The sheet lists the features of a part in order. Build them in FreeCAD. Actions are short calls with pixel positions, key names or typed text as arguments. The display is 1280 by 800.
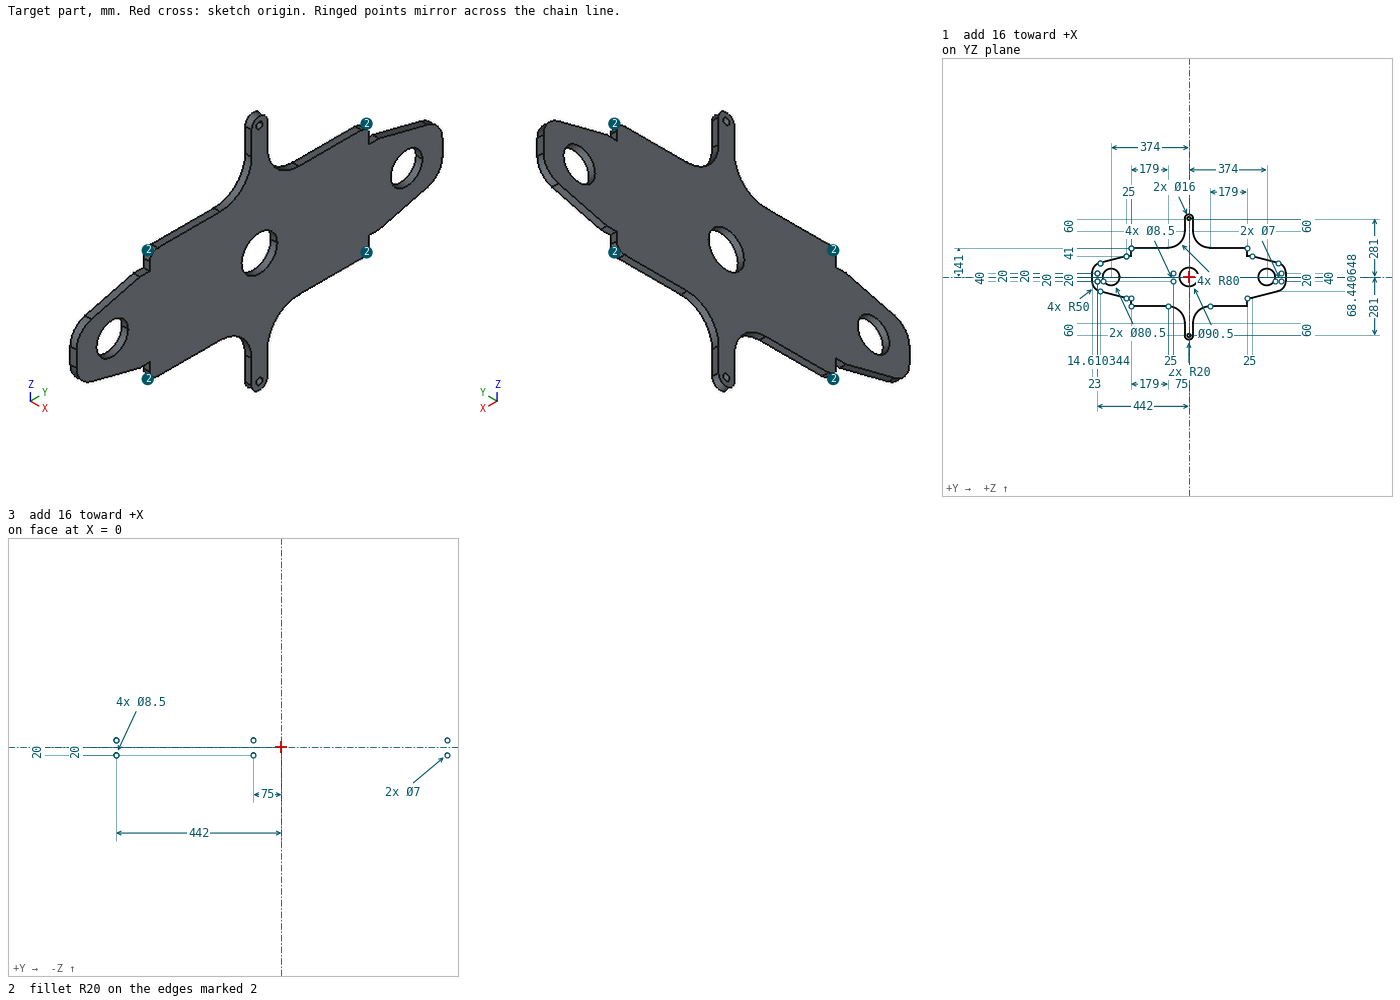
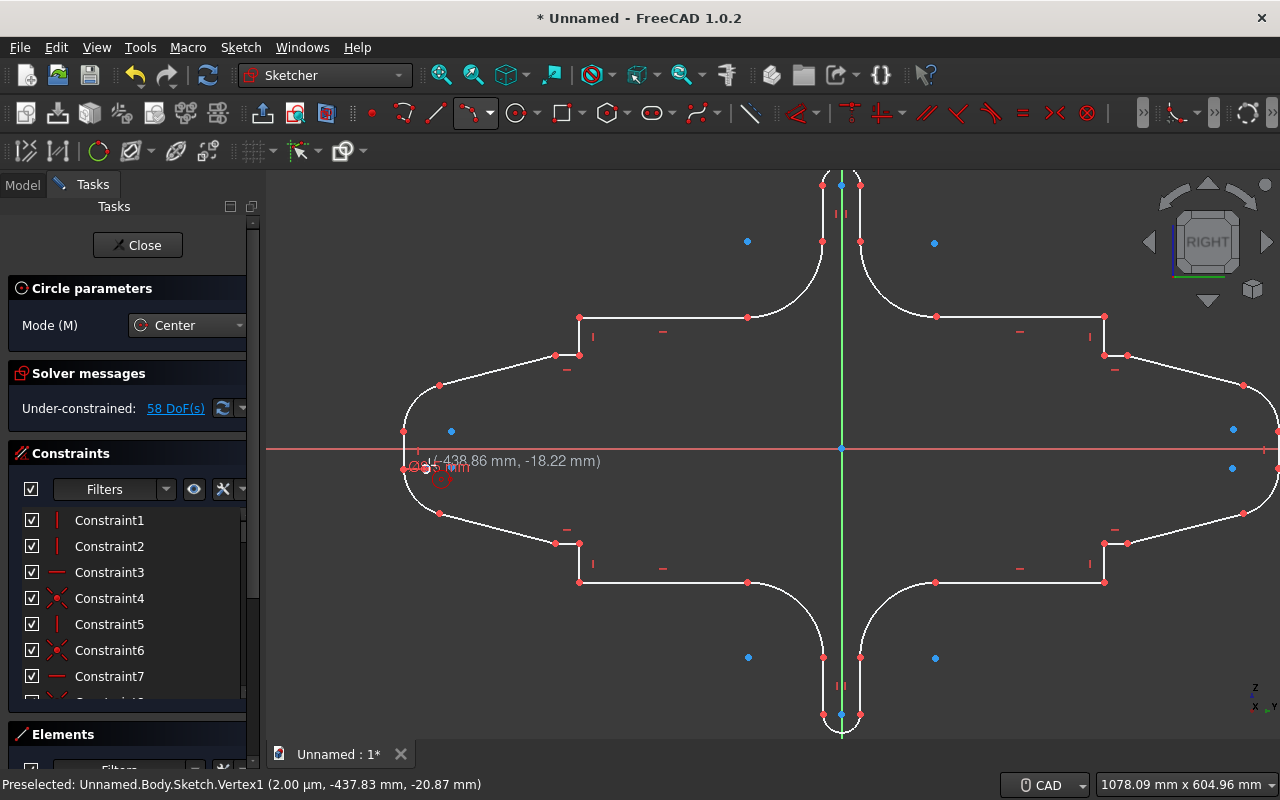
scroll(771, 468, up, 9)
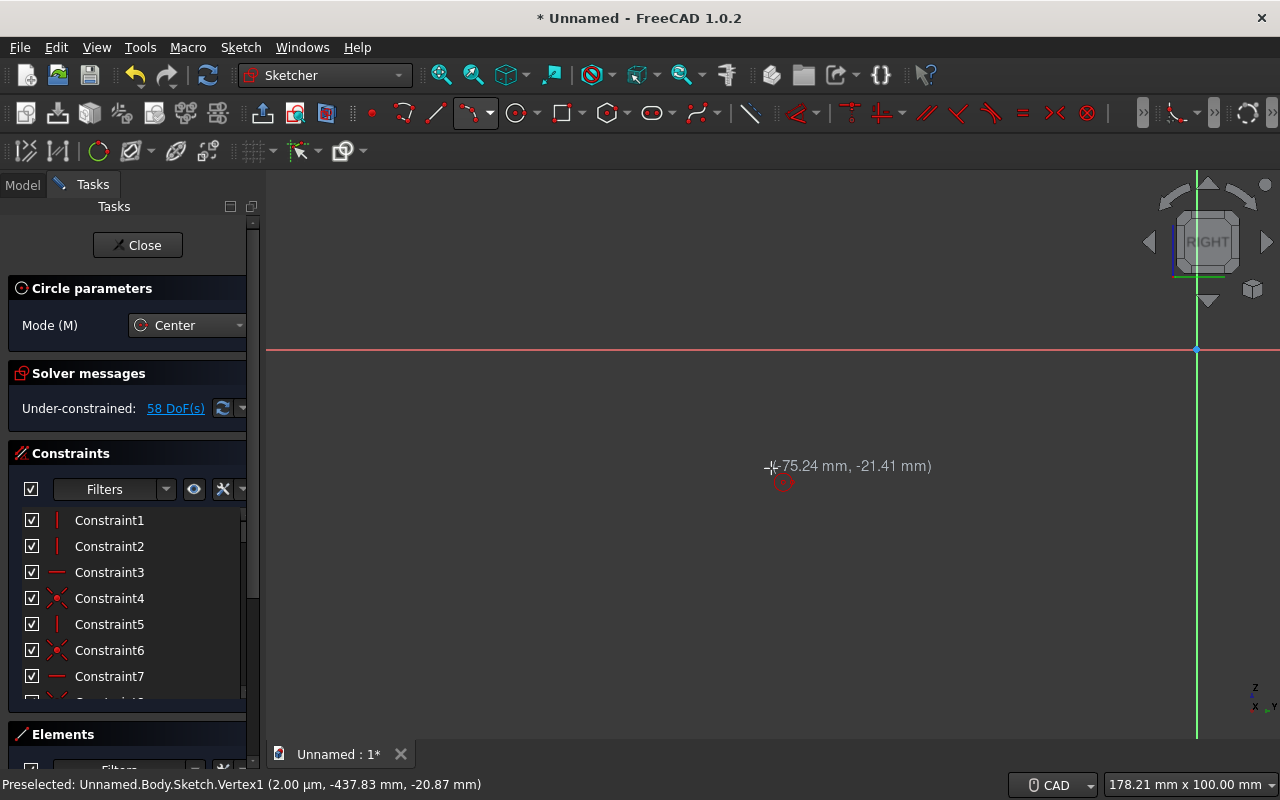
scroll(643, 468, down, 11)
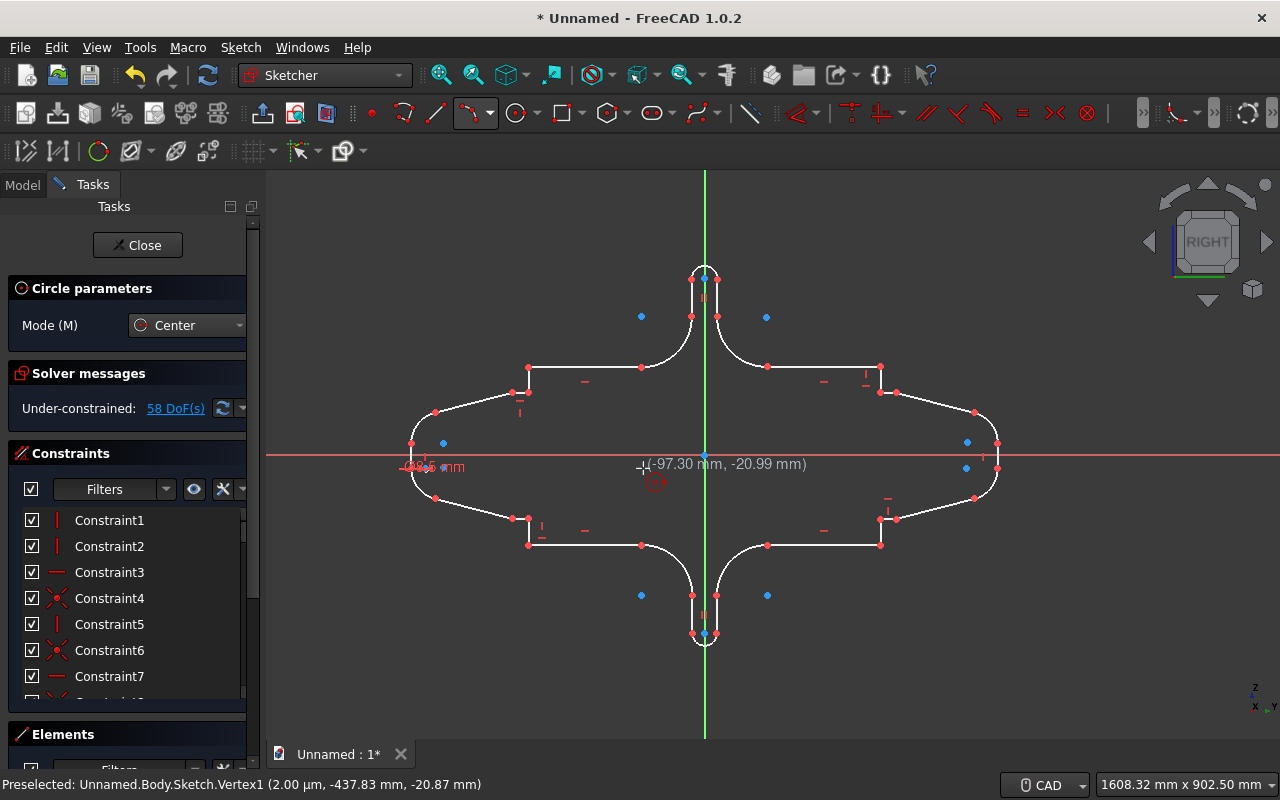
scroll(657, 468, up, 2)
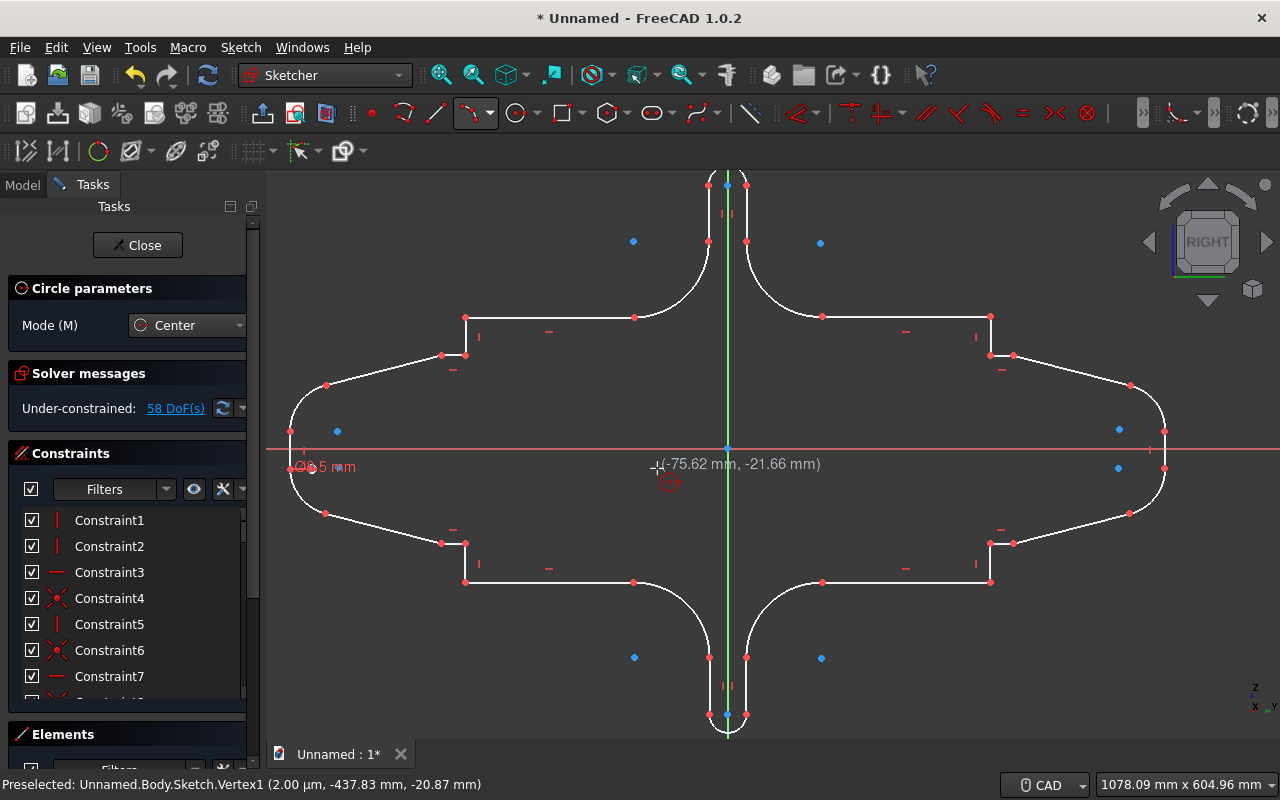
click(657, 468)
move(660, 465)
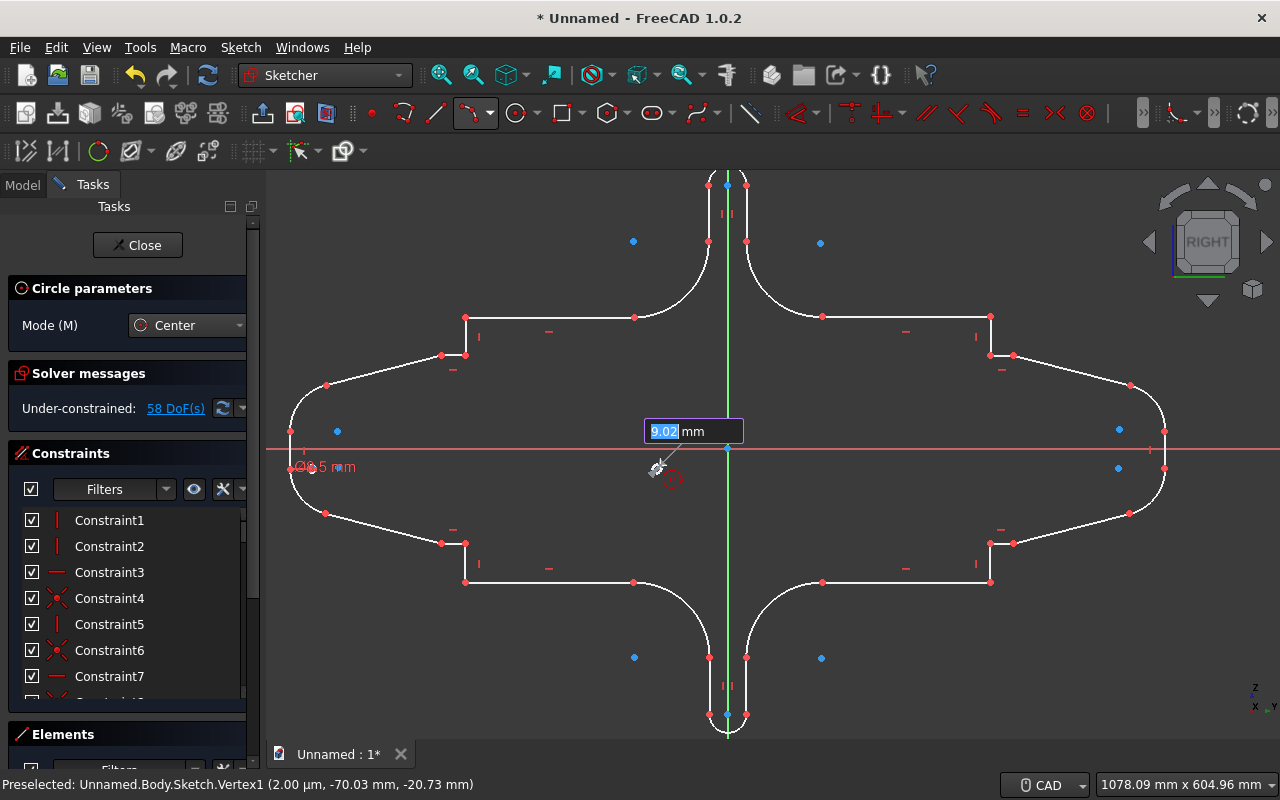
text(8.5)
key(Return)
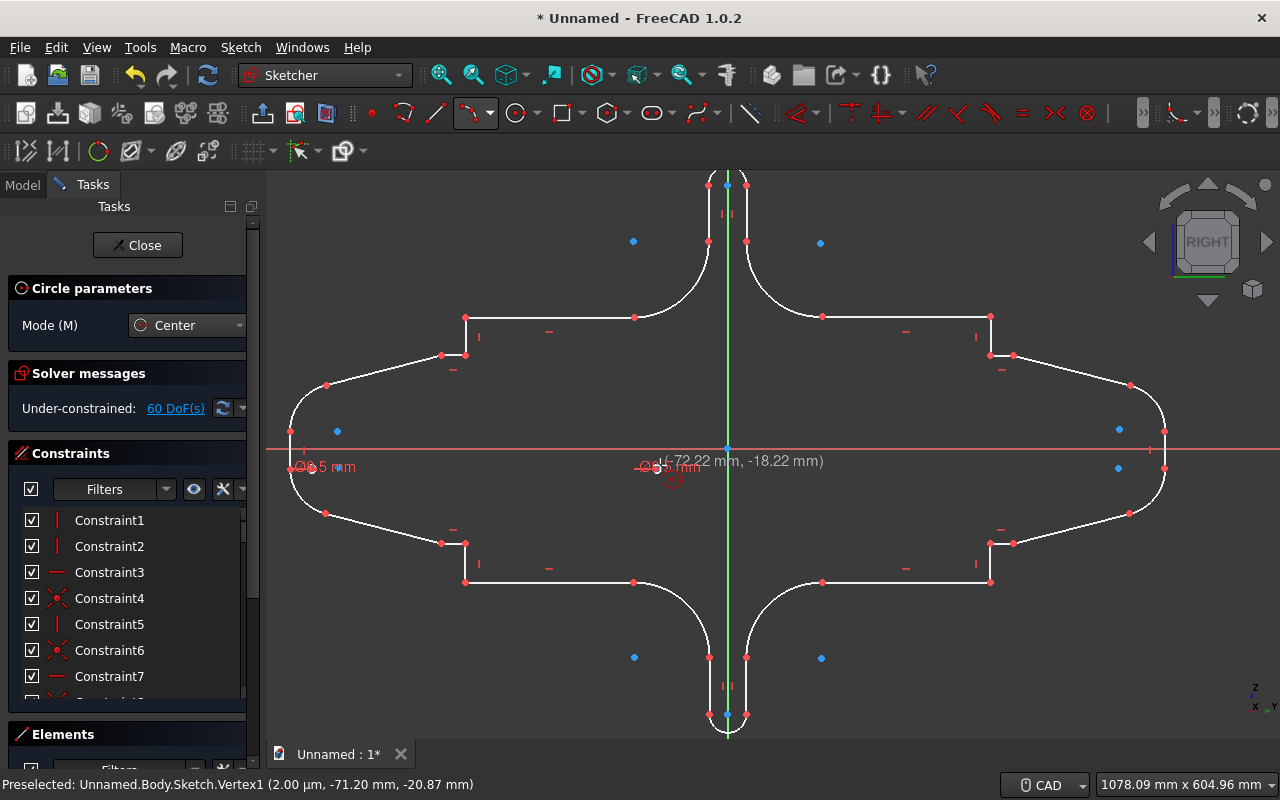
scroll(312, 430, up, 9)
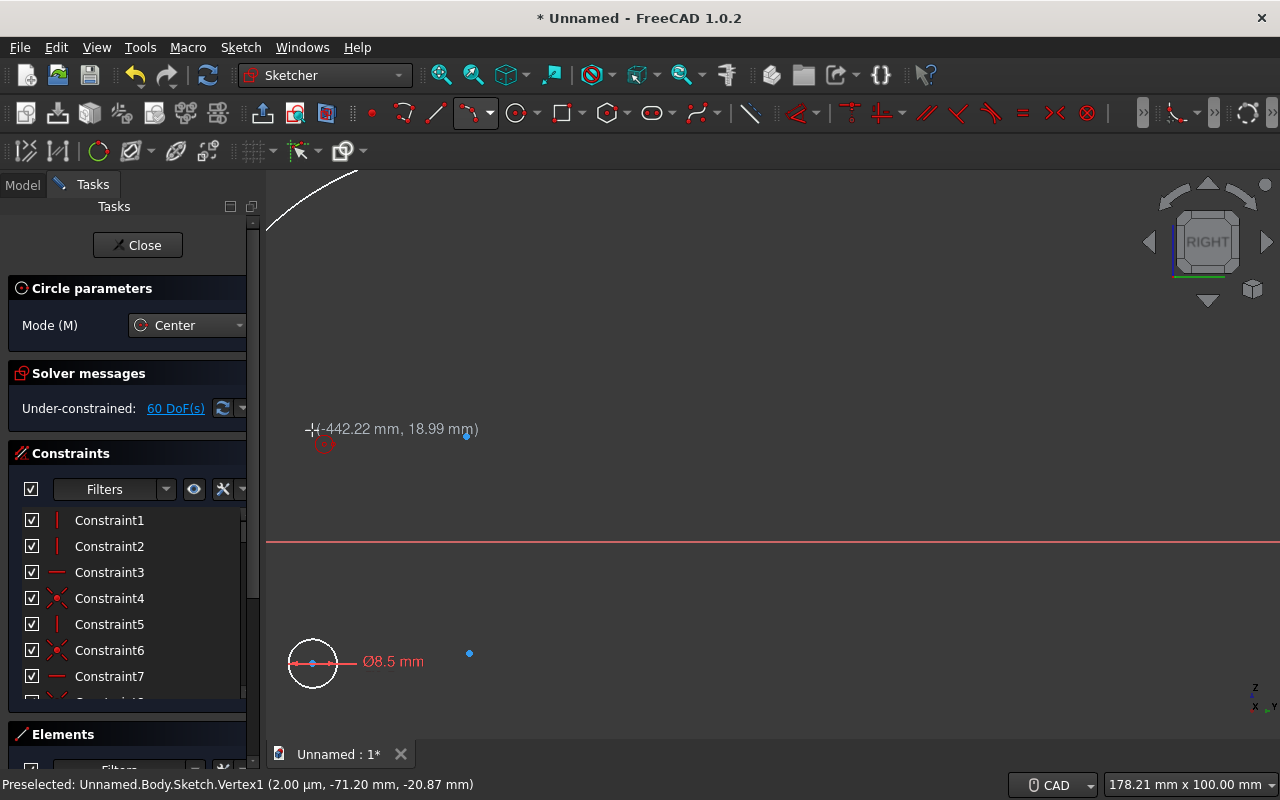
scroll(440, 444, down, 11)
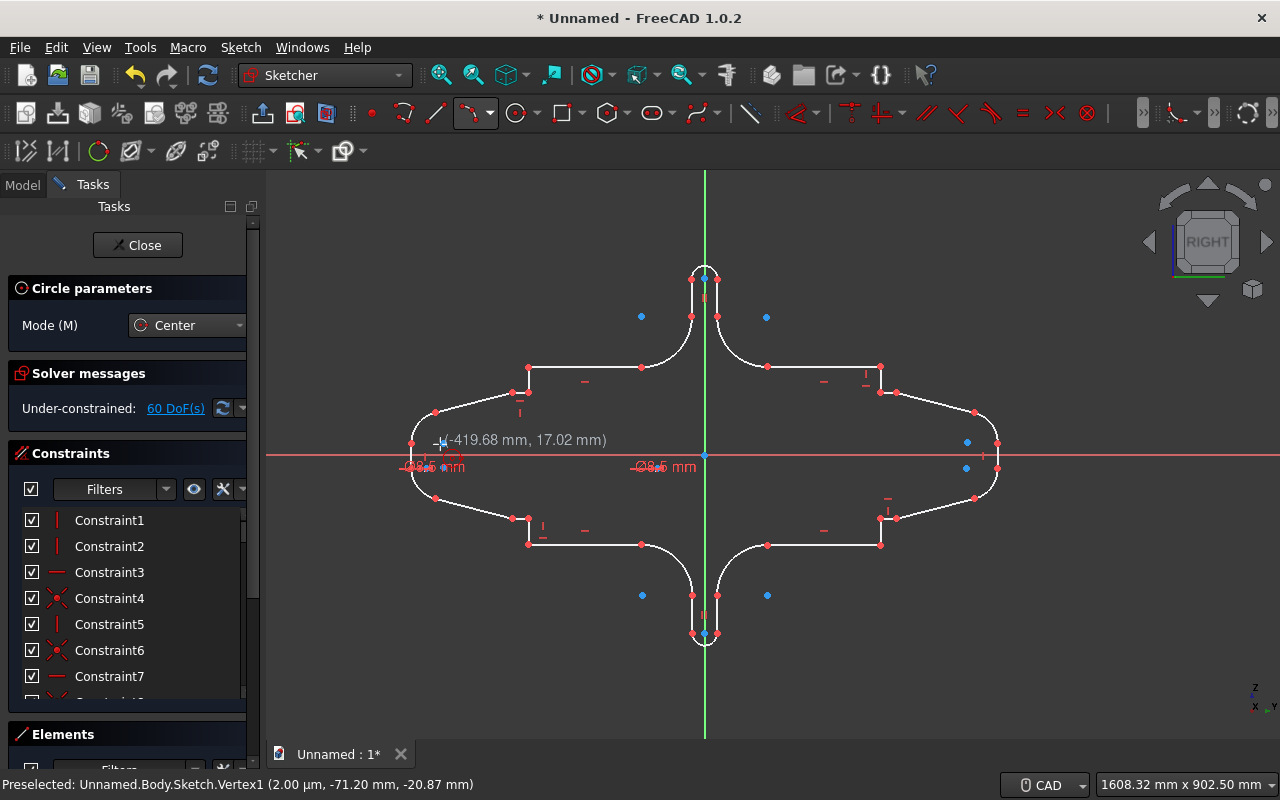
scroll(426, 443, up, 2)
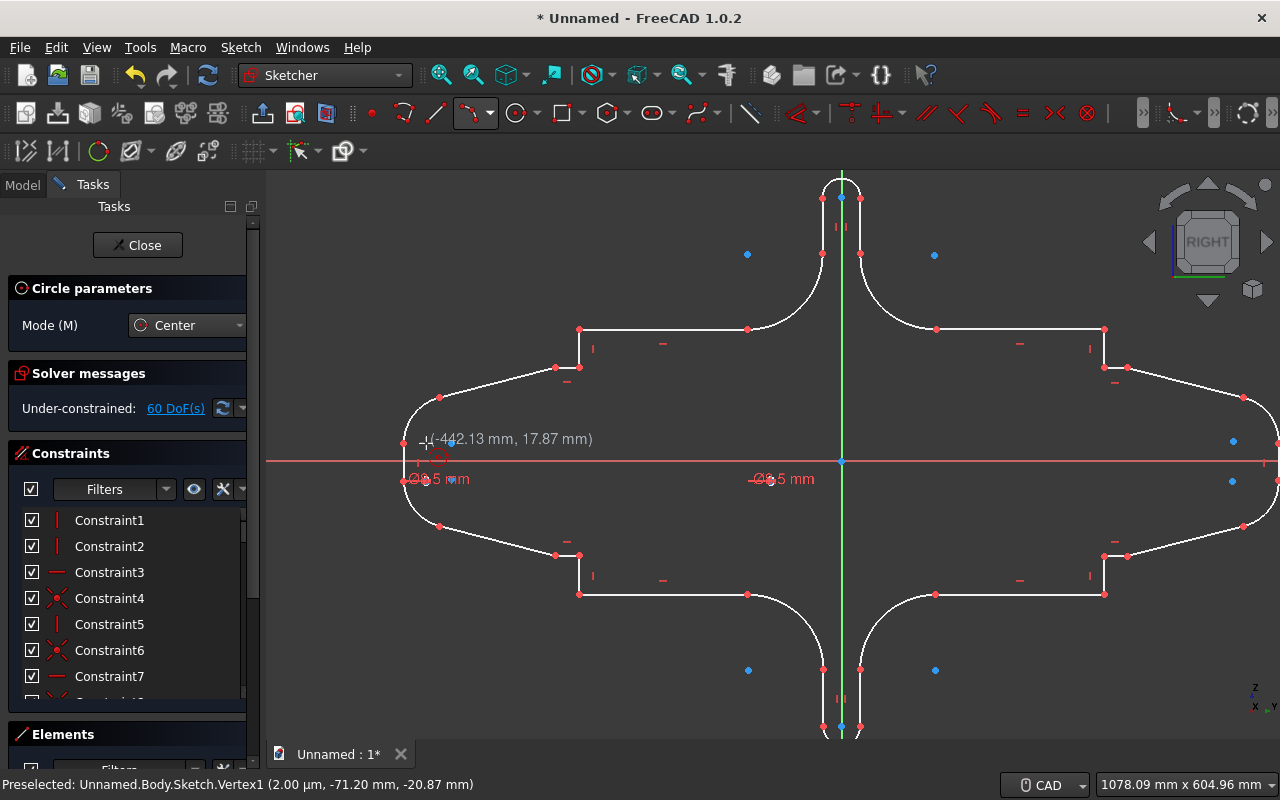
click(426, 442)
move(429, 439)